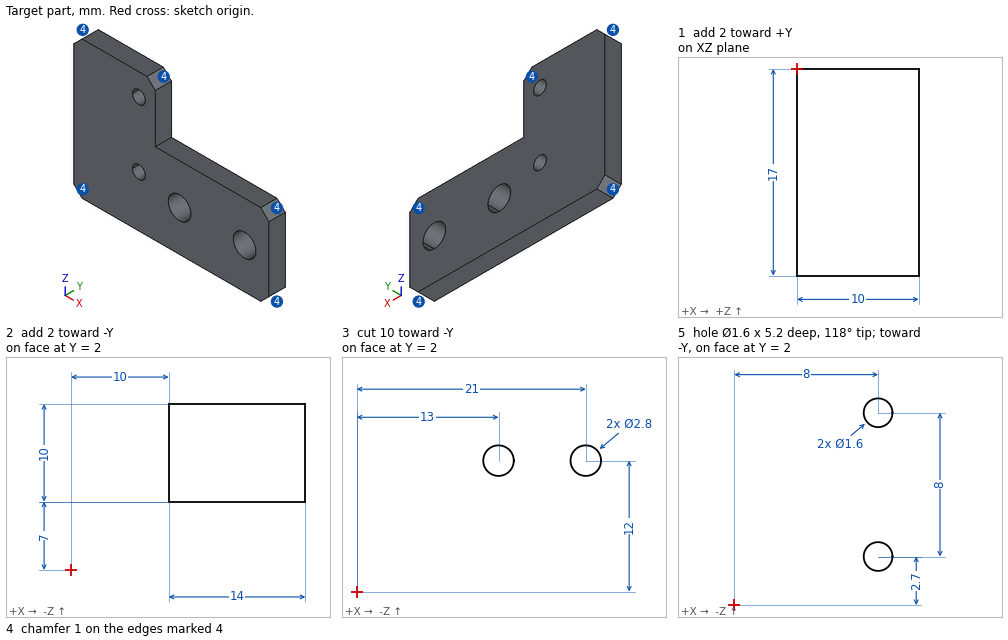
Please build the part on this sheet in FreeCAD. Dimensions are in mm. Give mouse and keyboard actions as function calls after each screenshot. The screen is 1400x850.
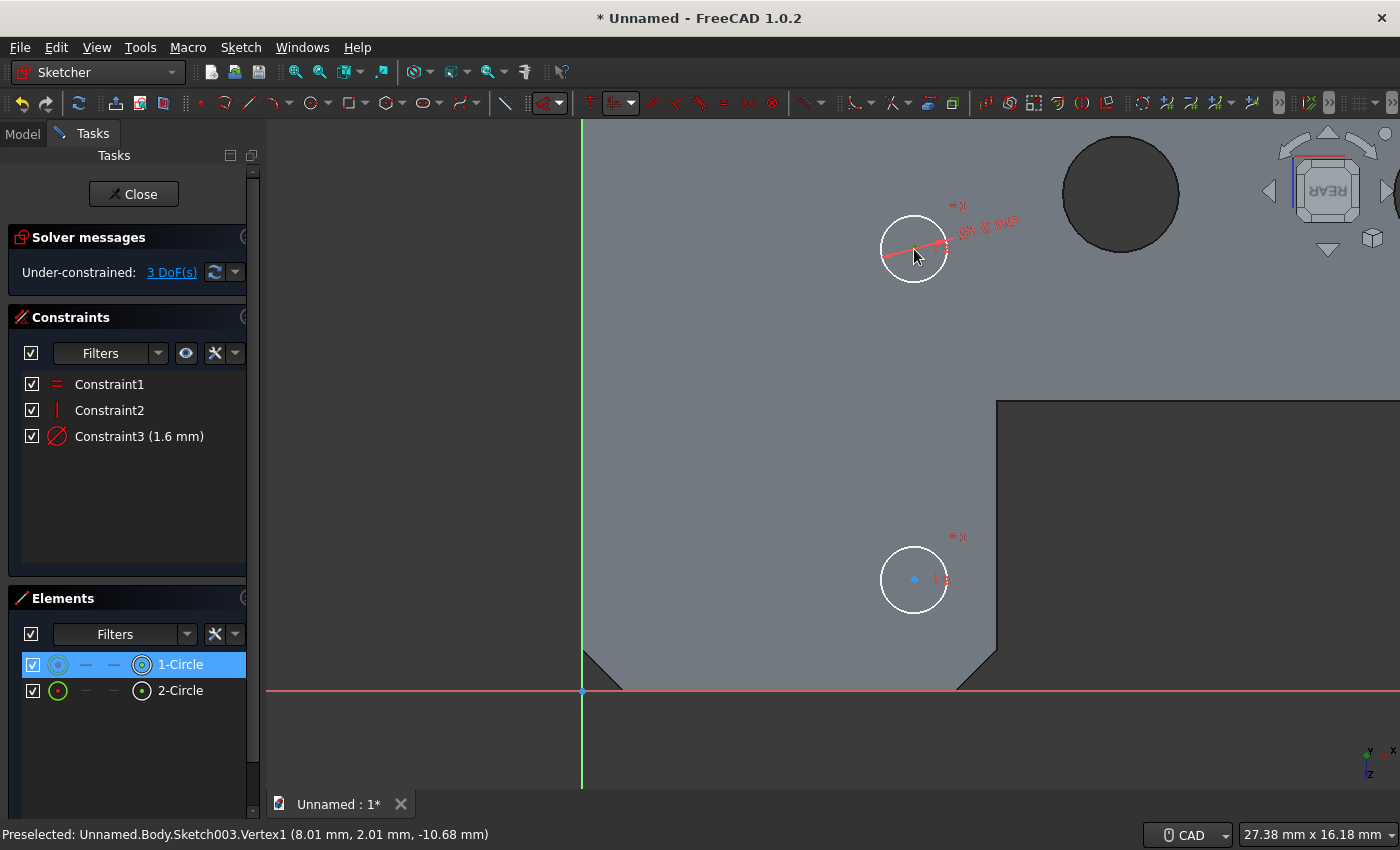
click(562, 104)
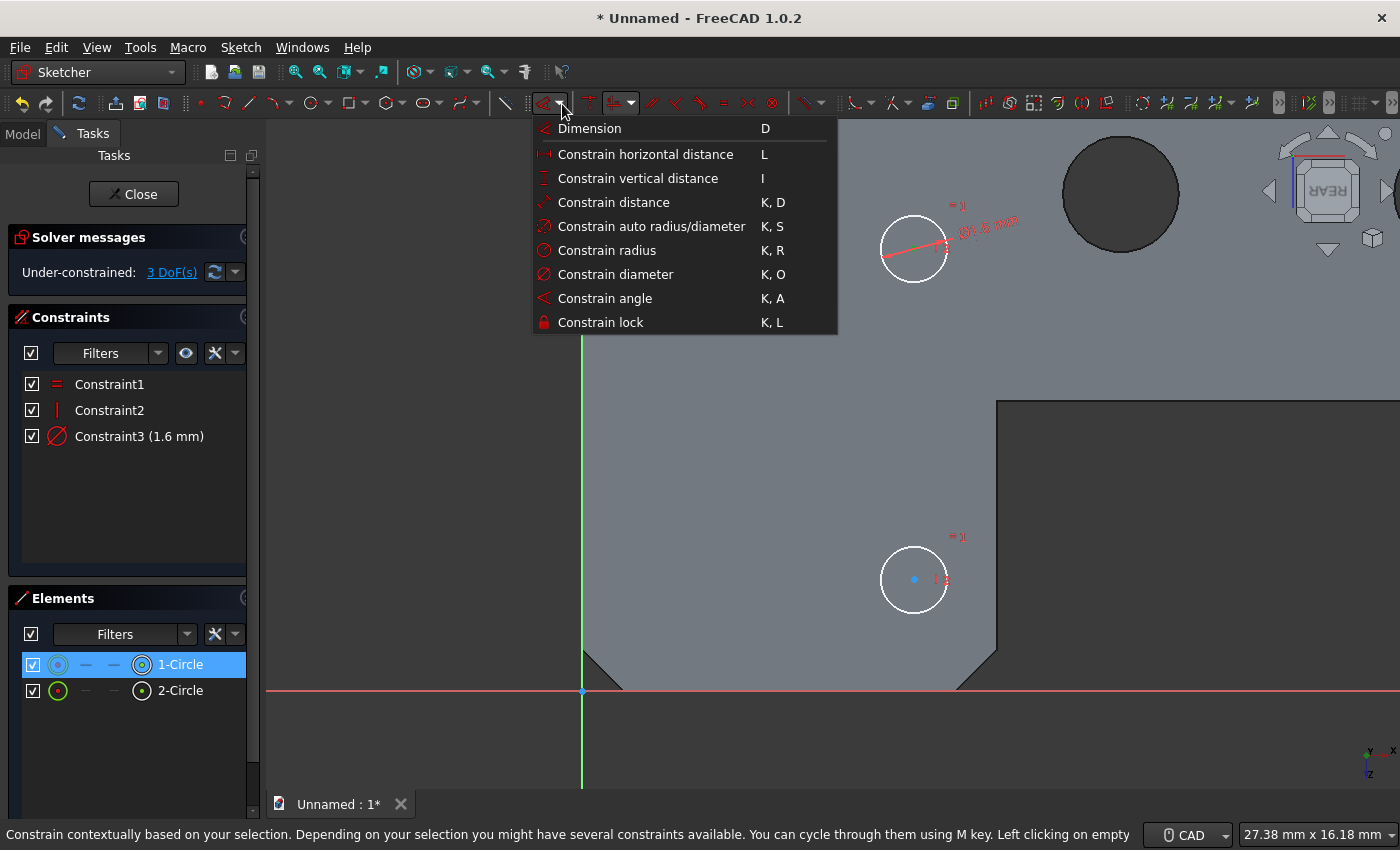
click(685, 154)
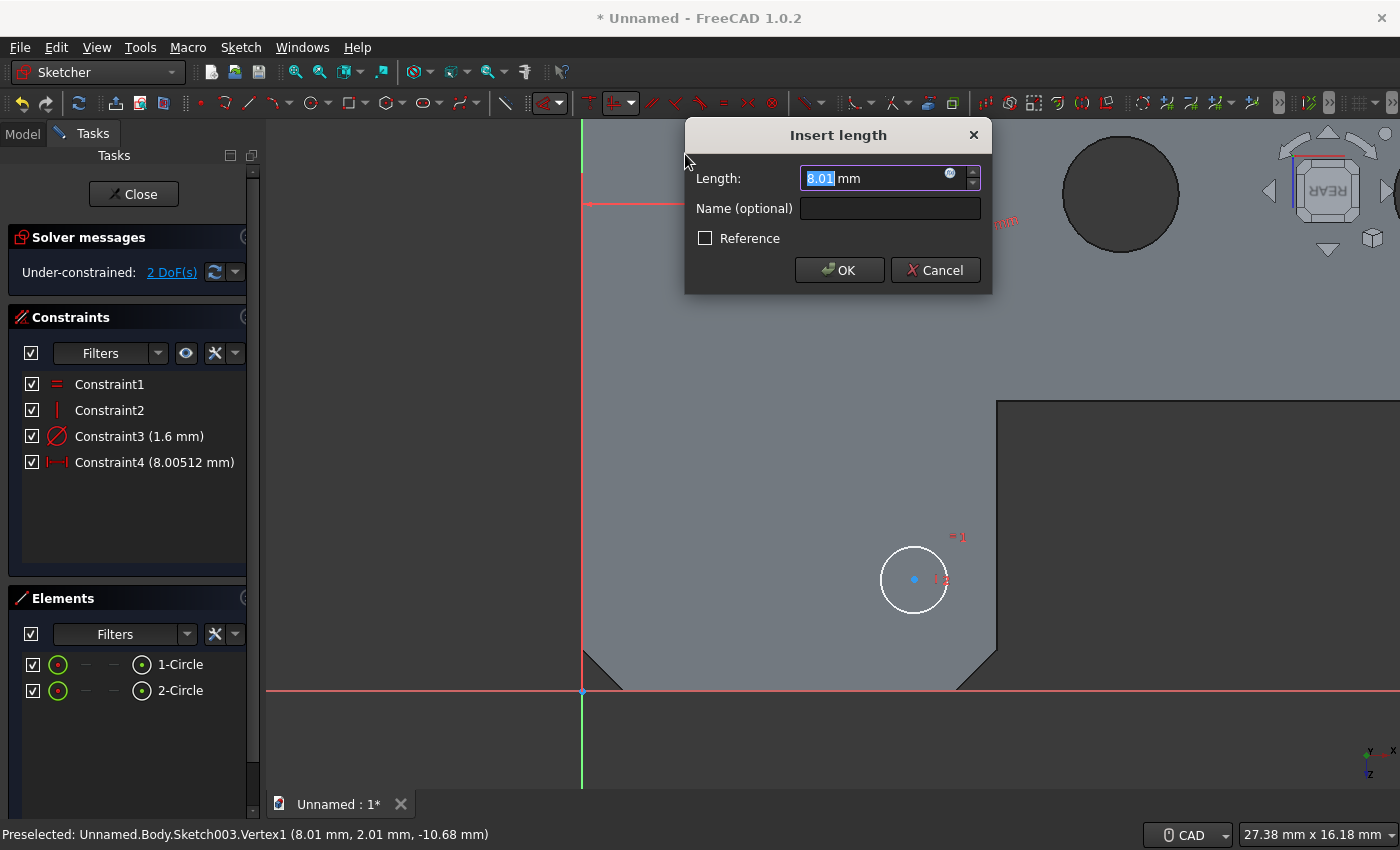
text(8)
key(Return)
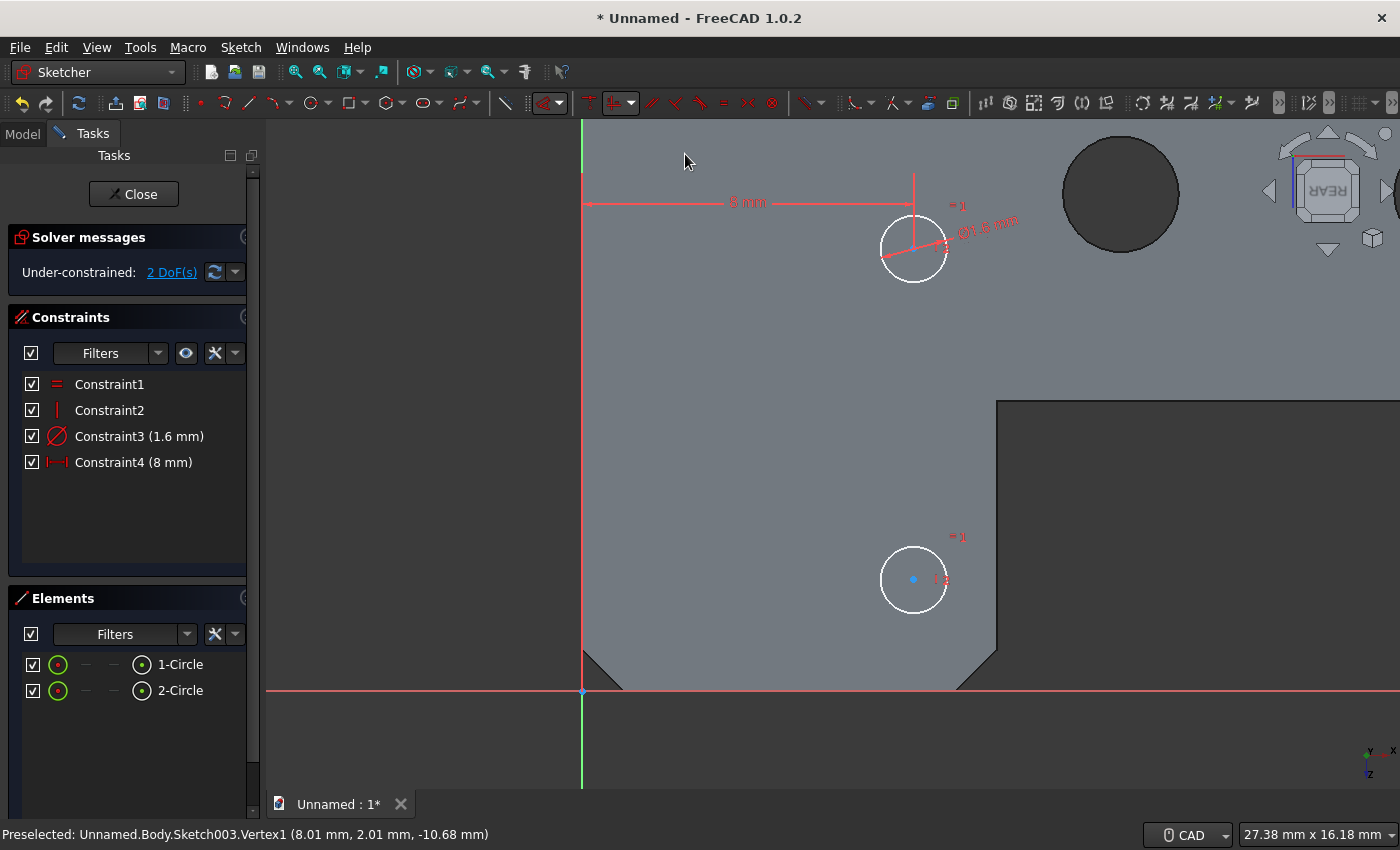
click(914, 249)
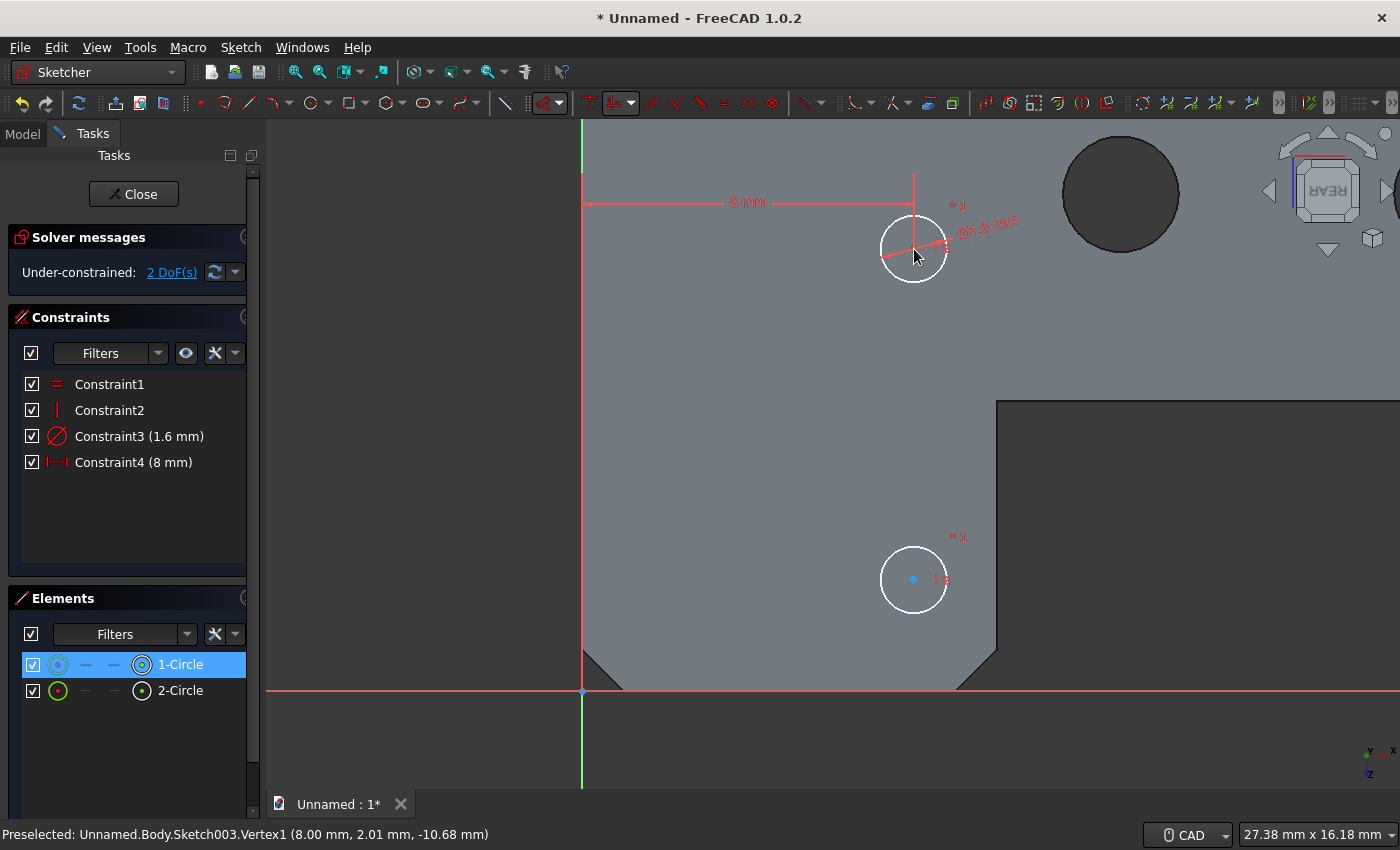
click(914, 580)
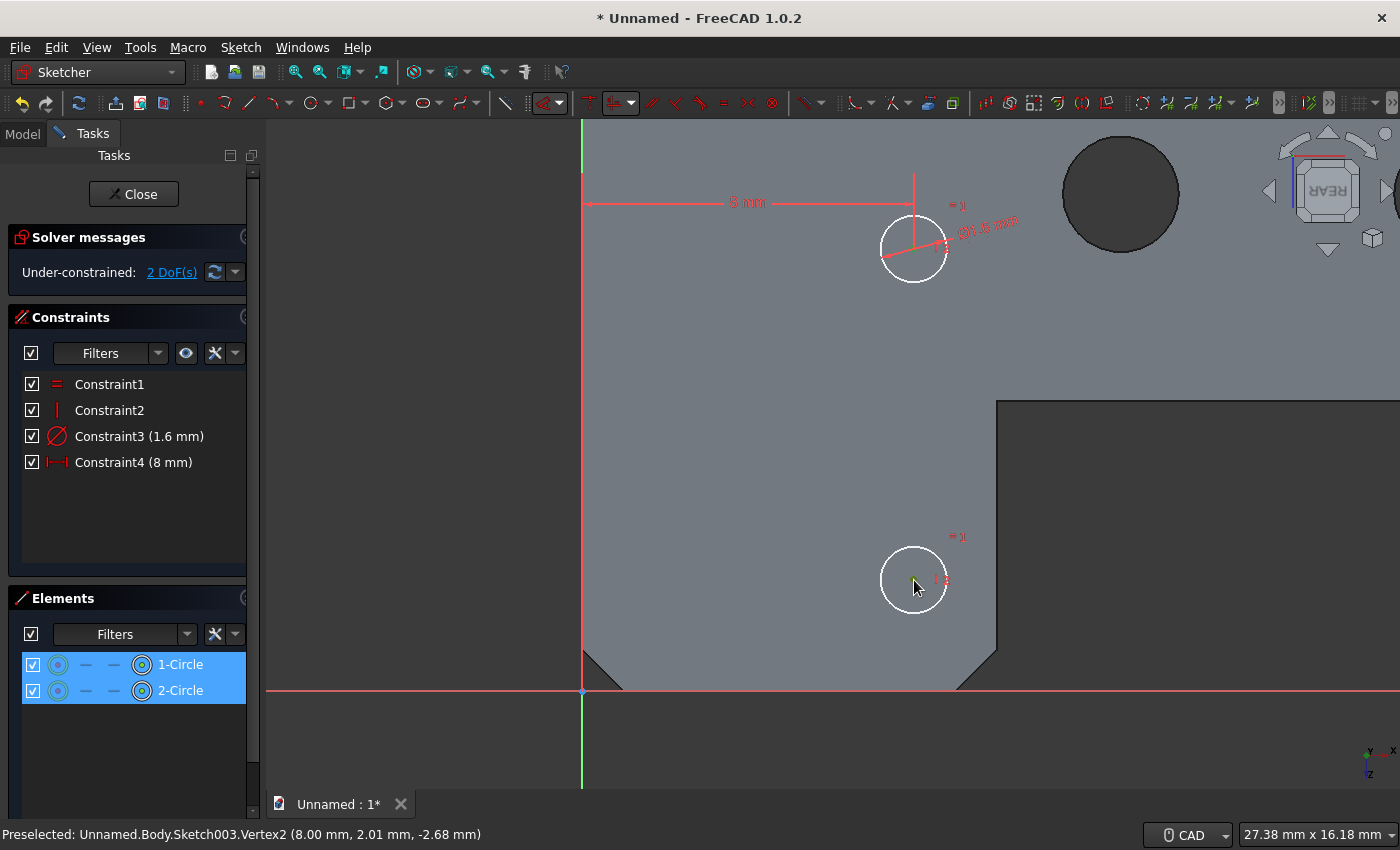
key(i)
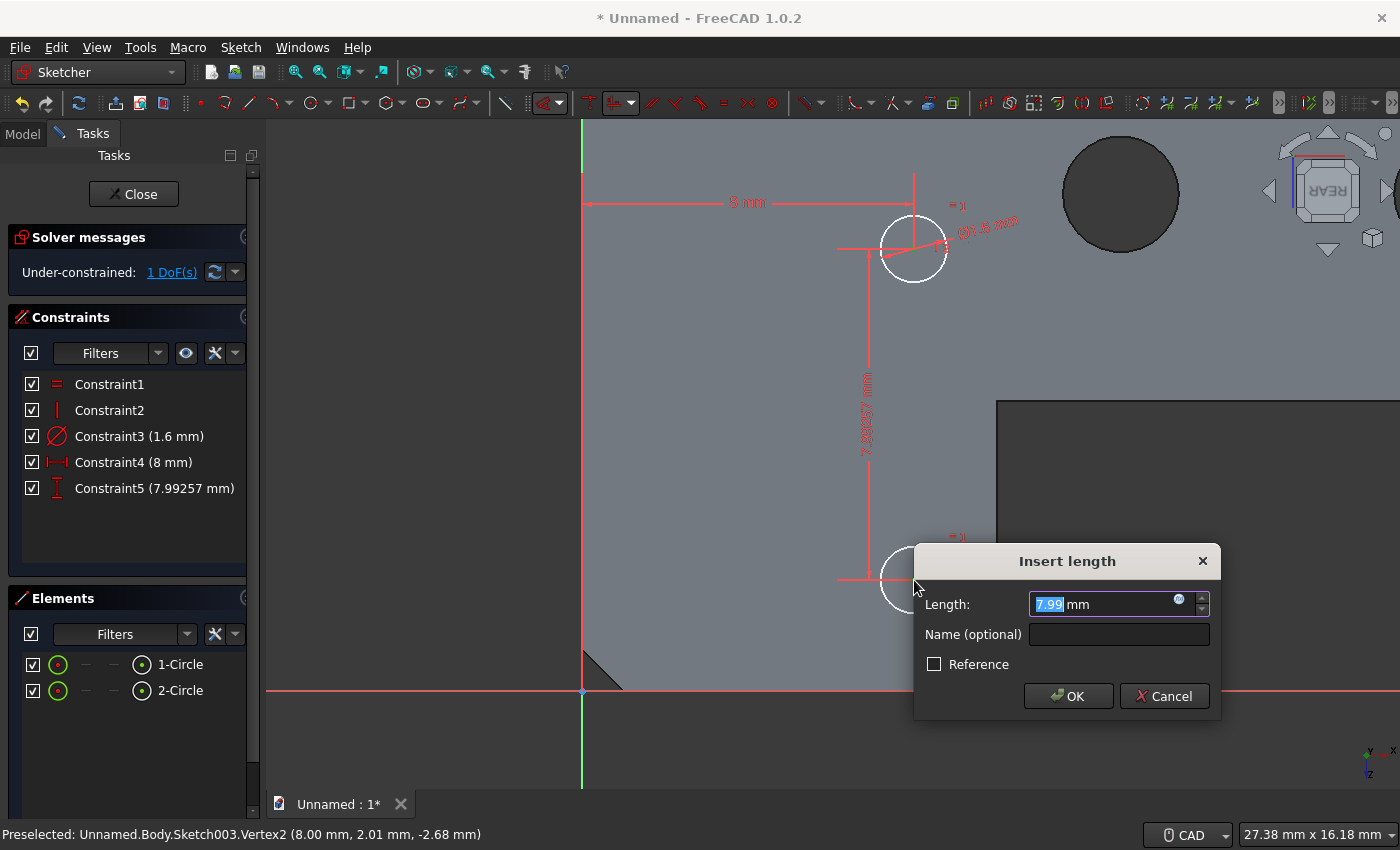
text(8)
key(Return)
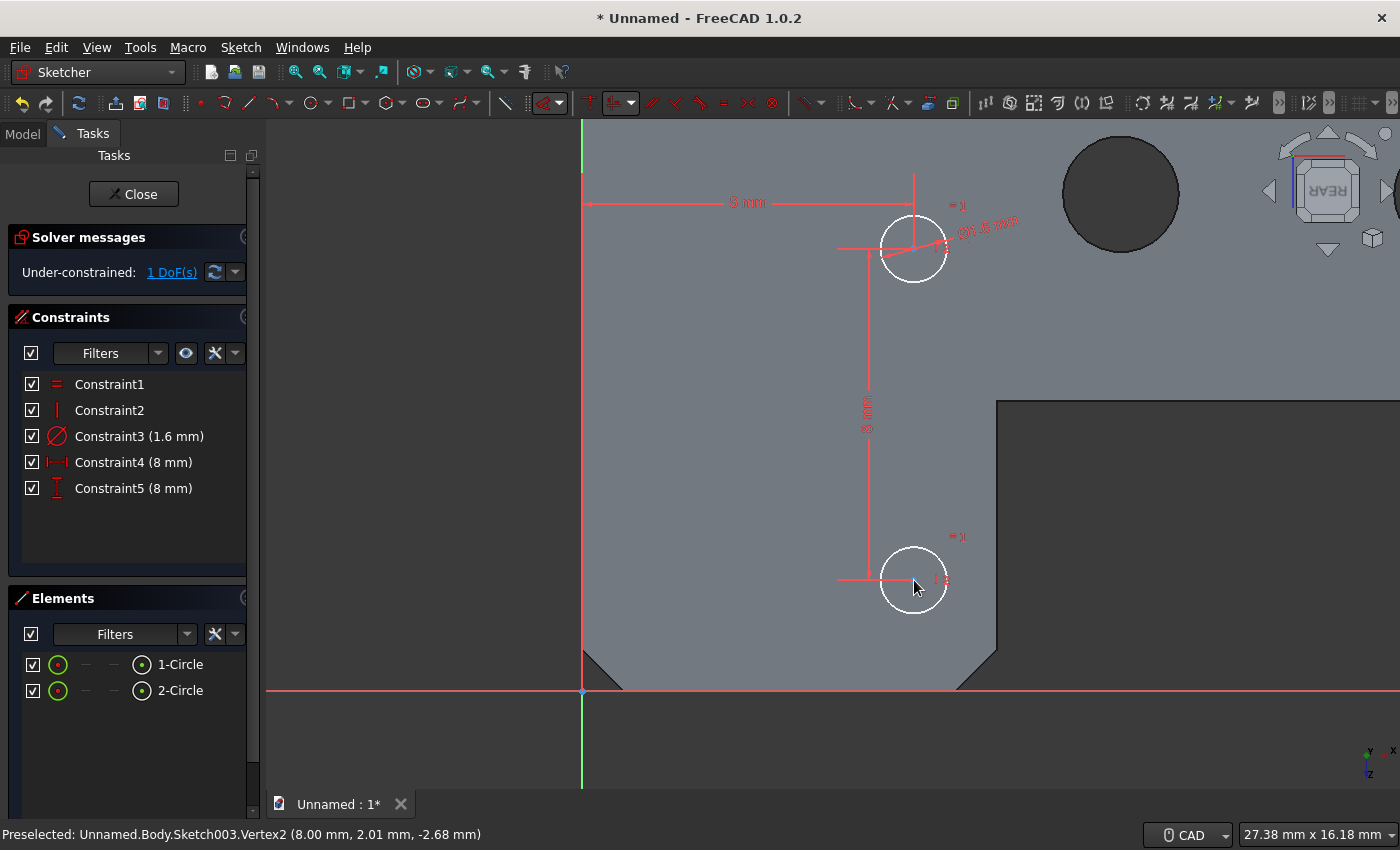
click(914, 580)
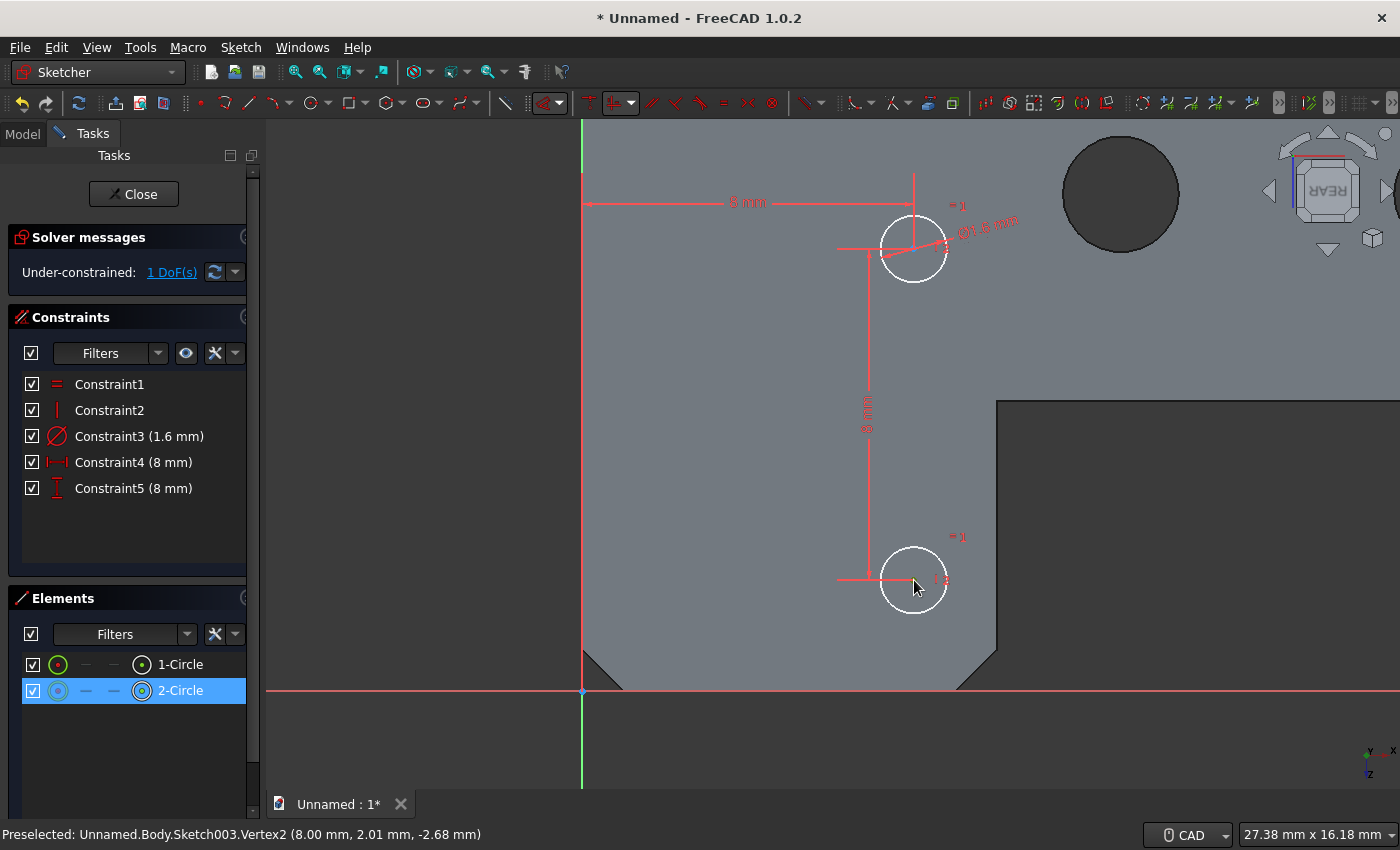
click(562, 104)